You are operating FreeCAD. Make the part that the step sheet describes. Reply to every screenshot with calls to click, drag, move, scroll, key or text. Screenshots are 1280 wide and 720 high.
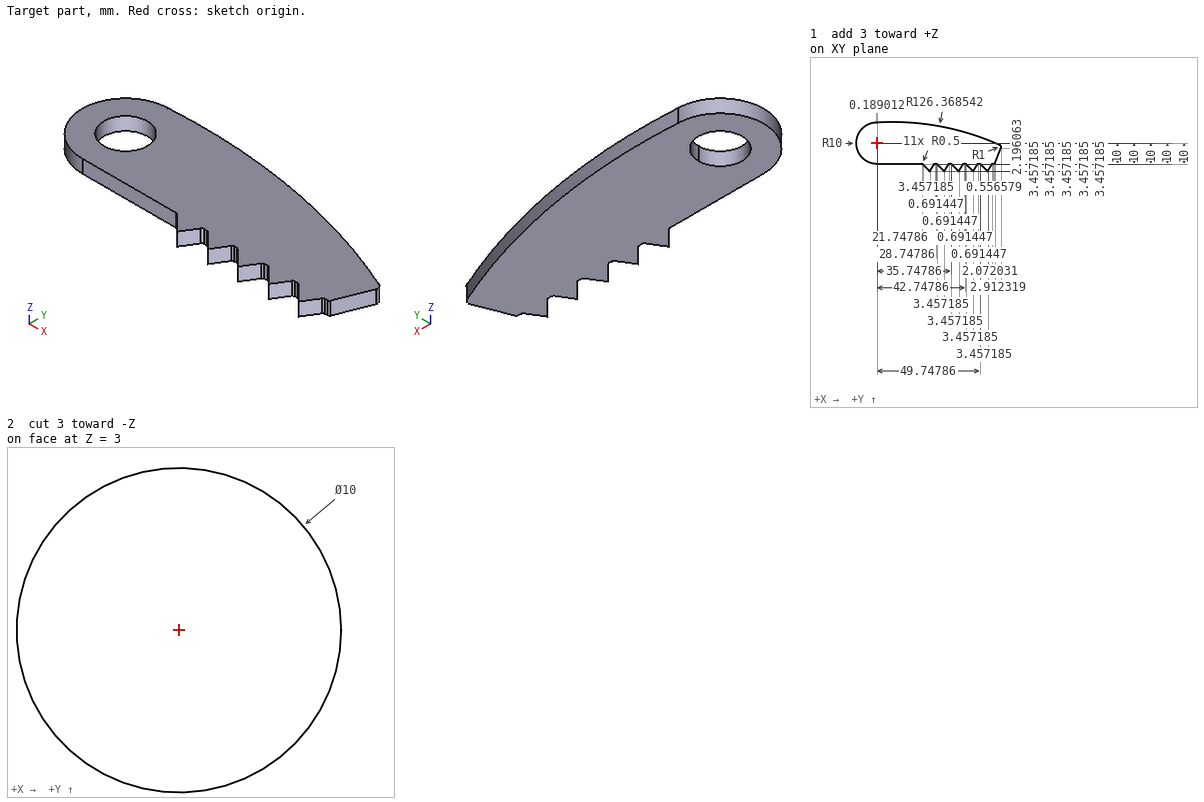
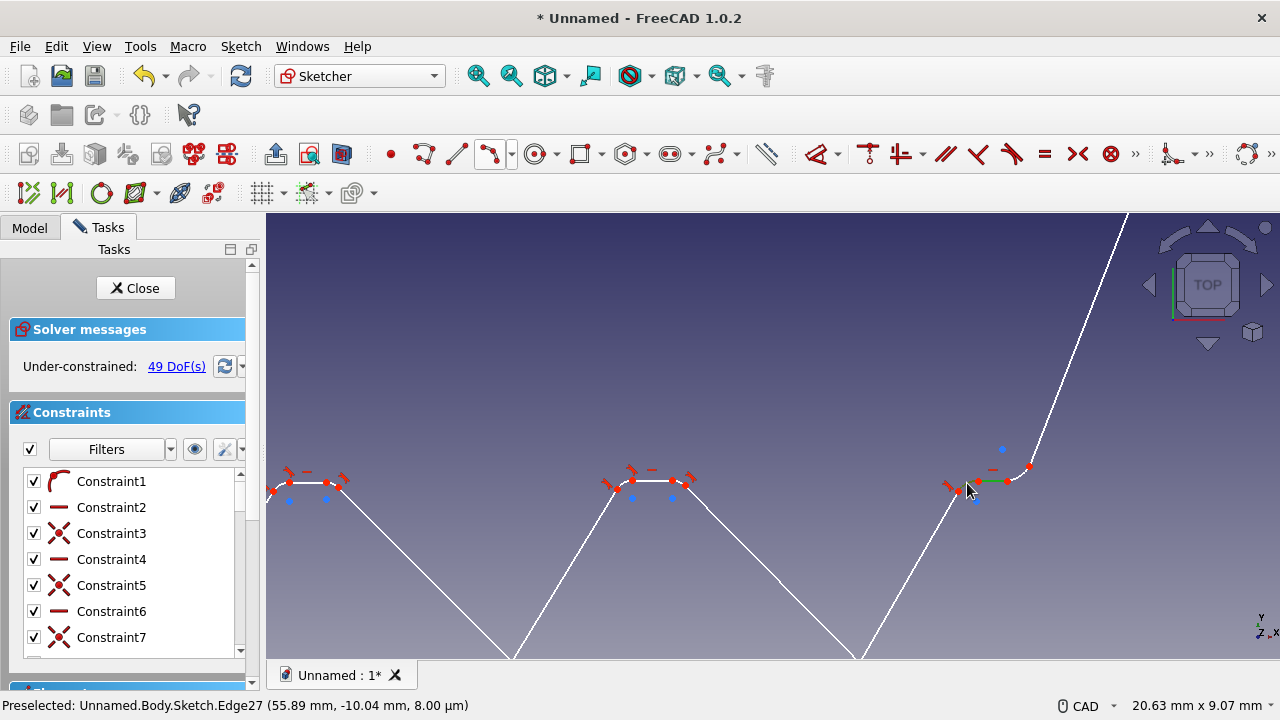
click(1012, 154)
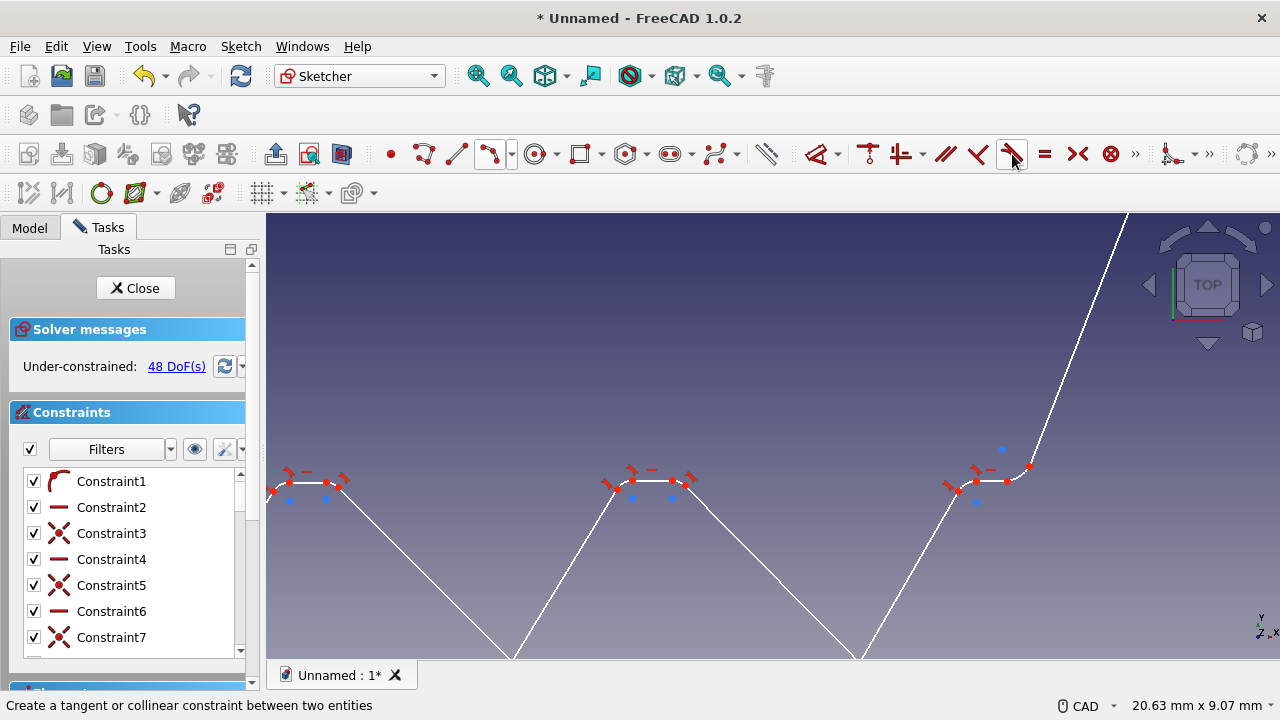
scroll(986, 481, up, 3)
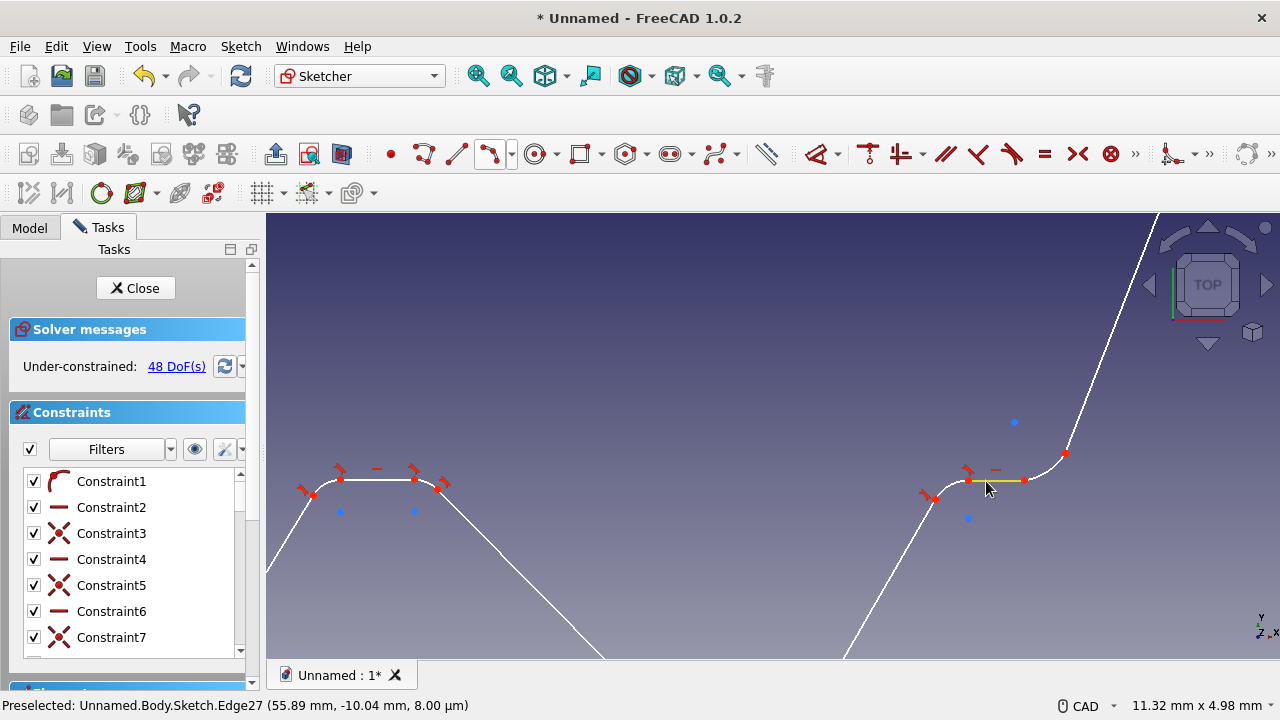
click(985, 481)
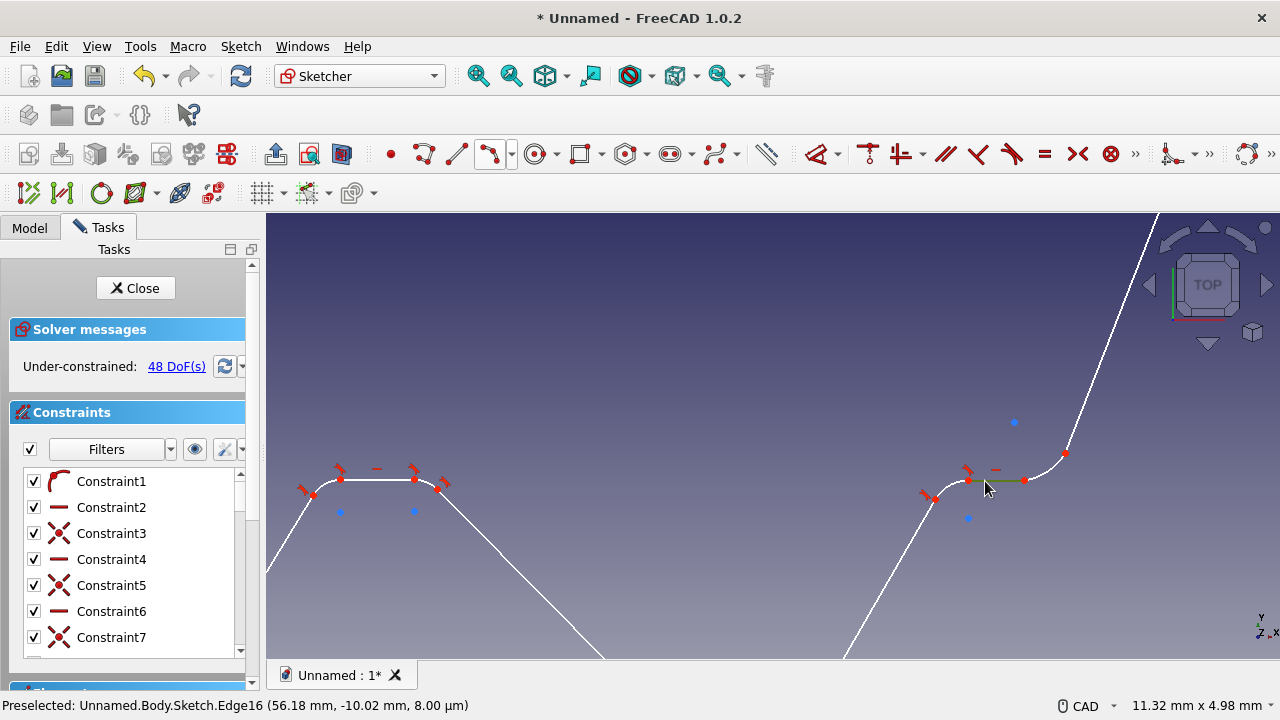
click(1039, 476)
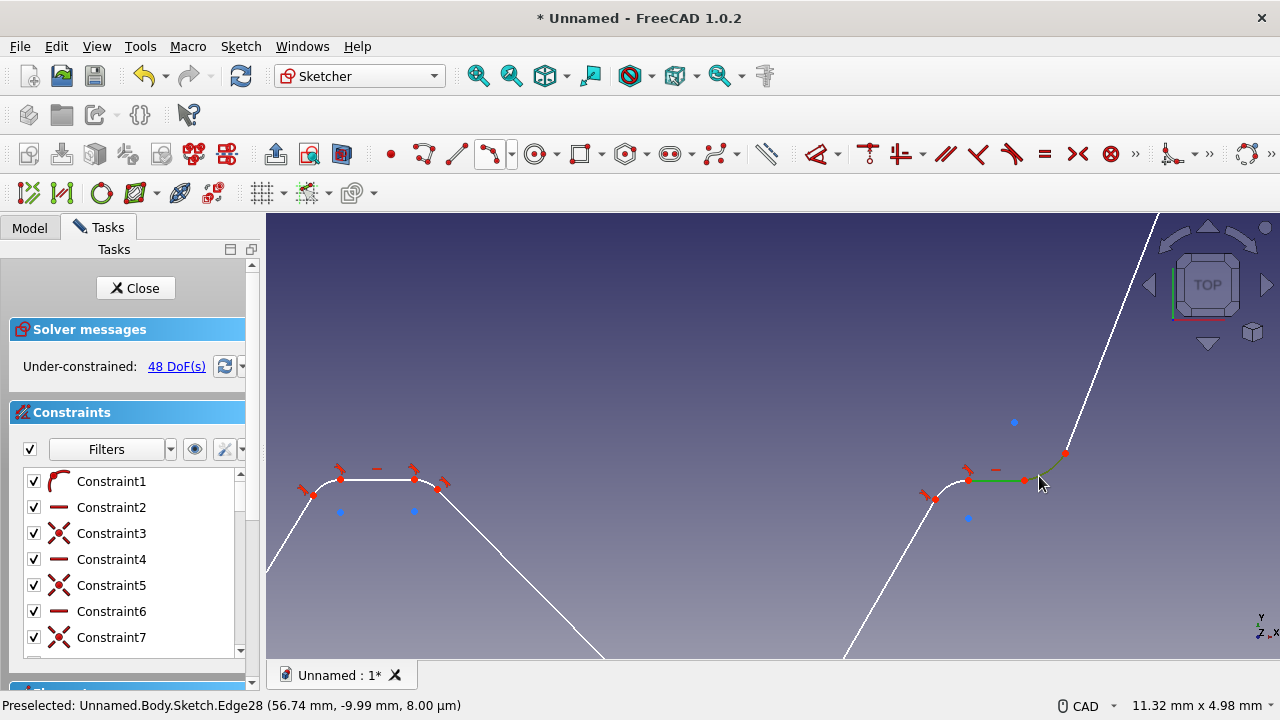
click(1012, 154)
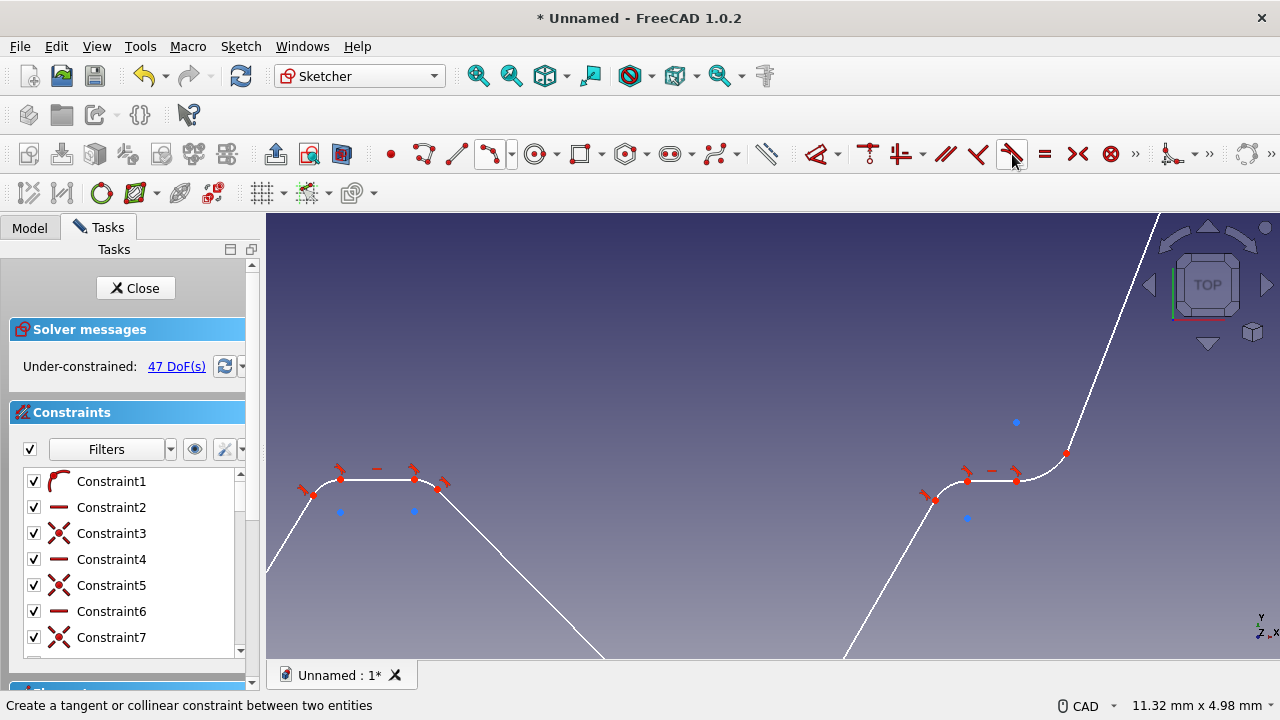
scroll(955, 505, down, 12)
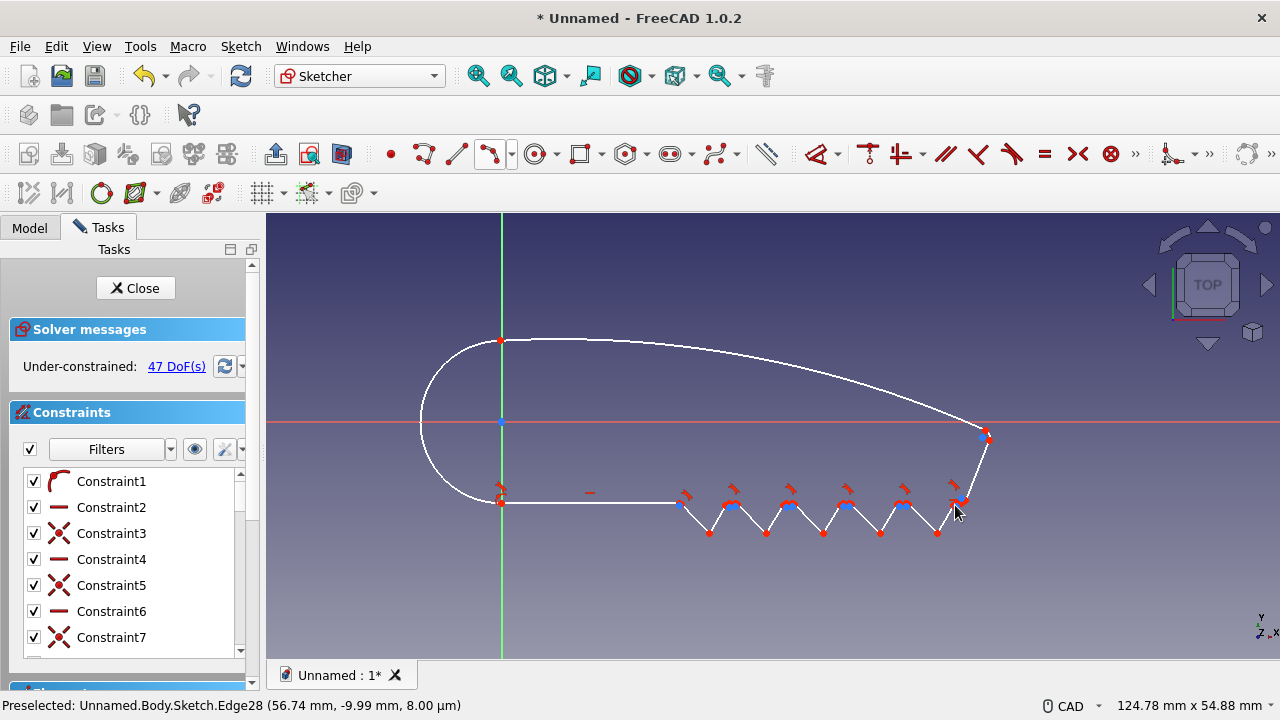
click(982, 459)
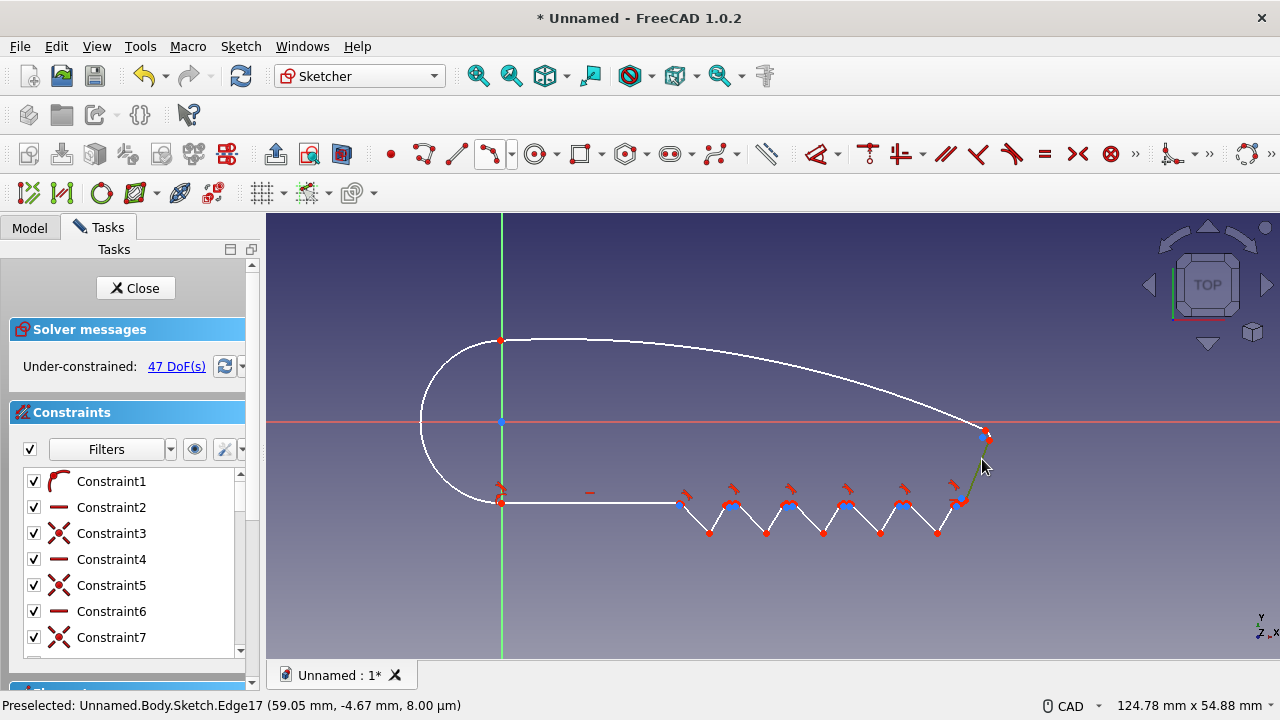
scroll(964, 503, up, 9)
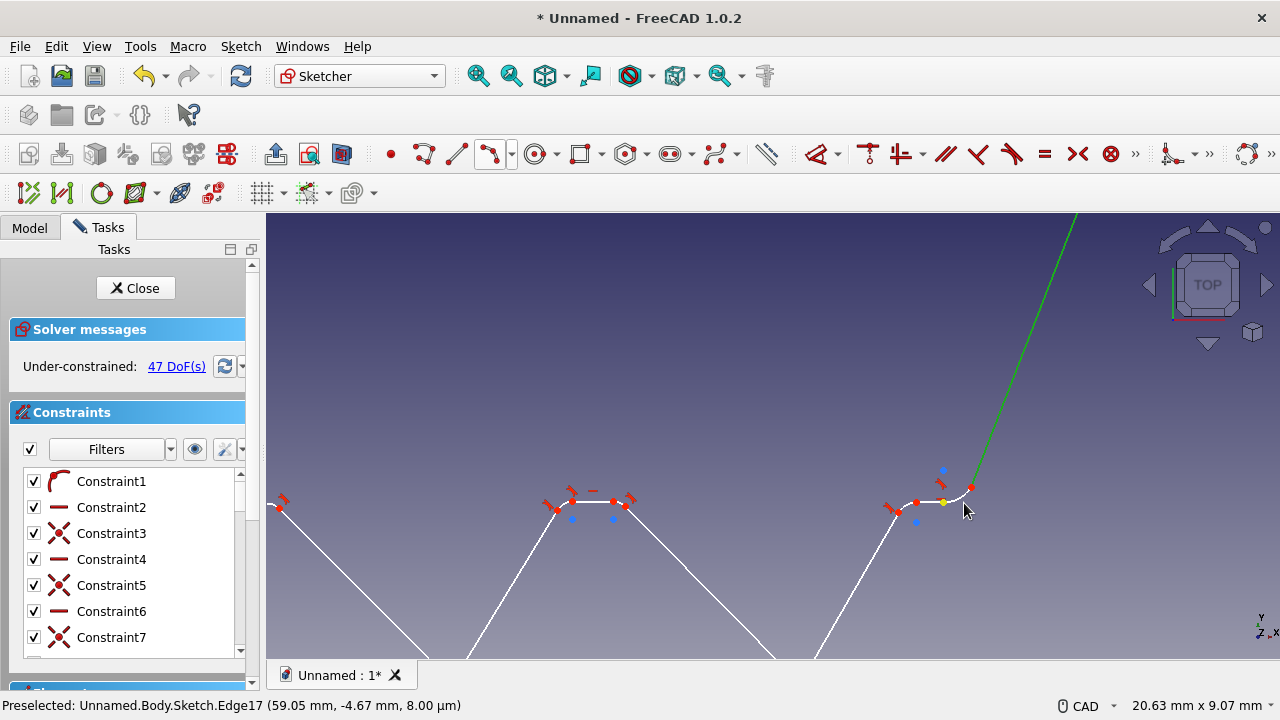
click(959, 498)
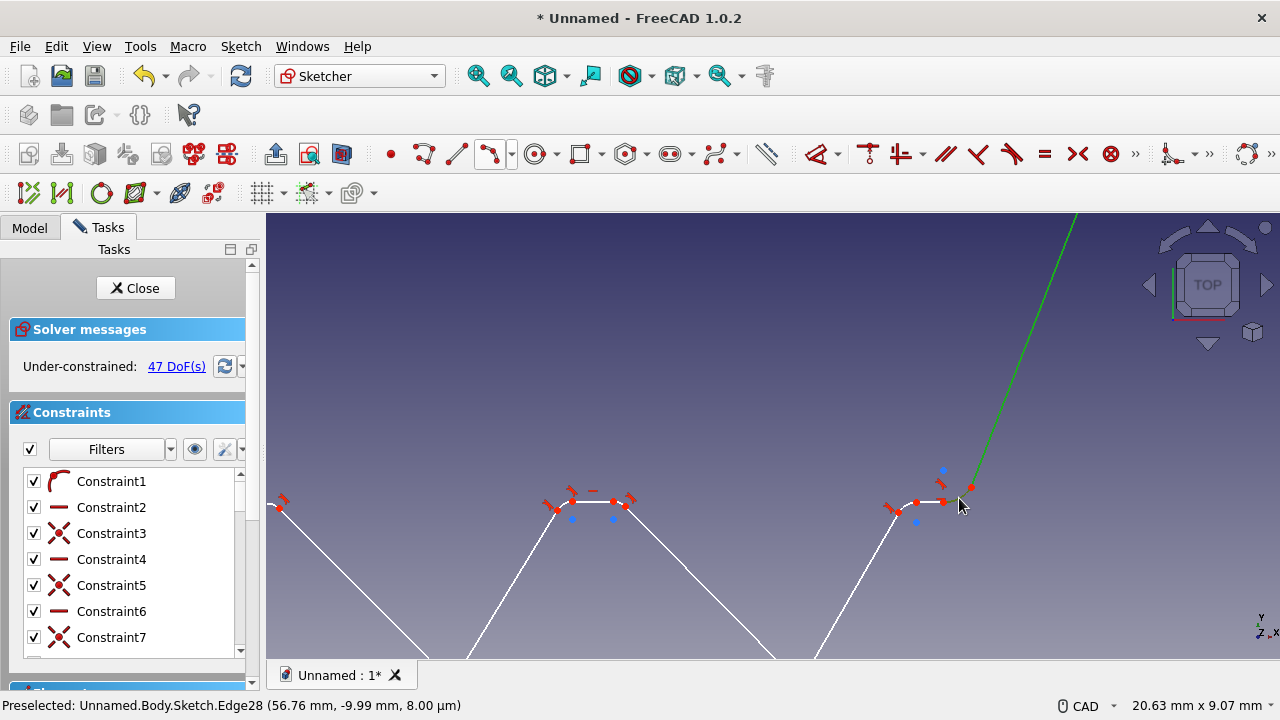
click(1012, 154)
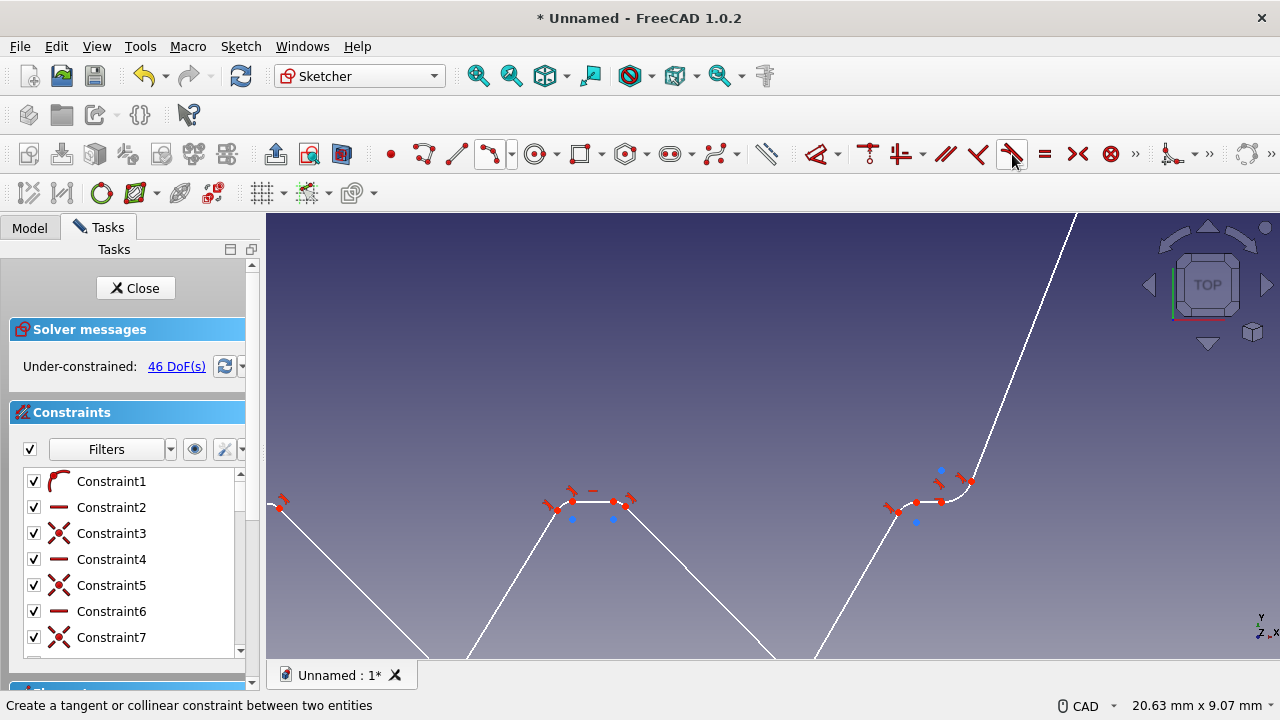
scroll(964, 503, down, 9)